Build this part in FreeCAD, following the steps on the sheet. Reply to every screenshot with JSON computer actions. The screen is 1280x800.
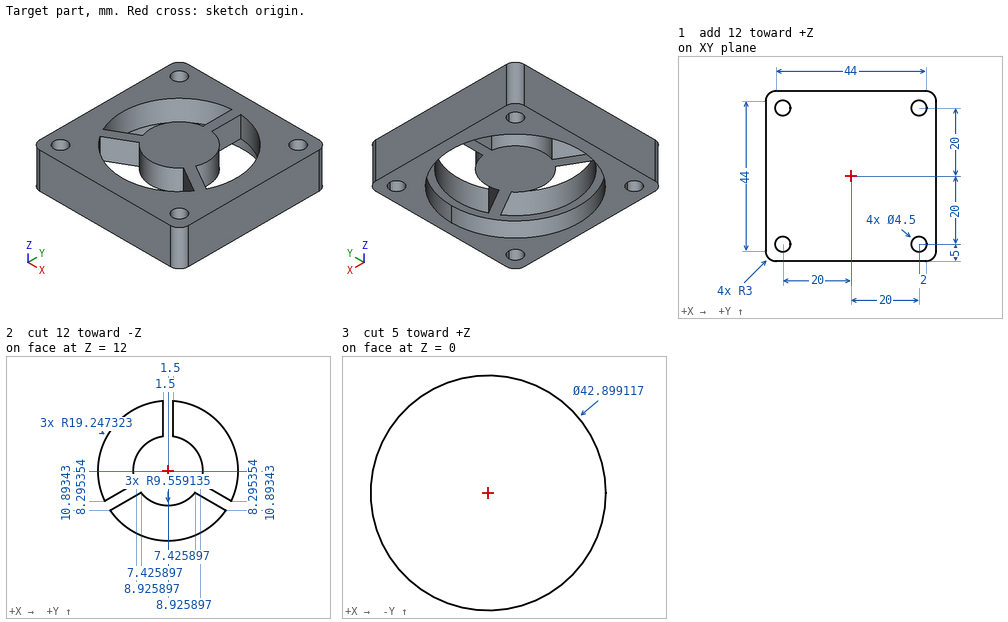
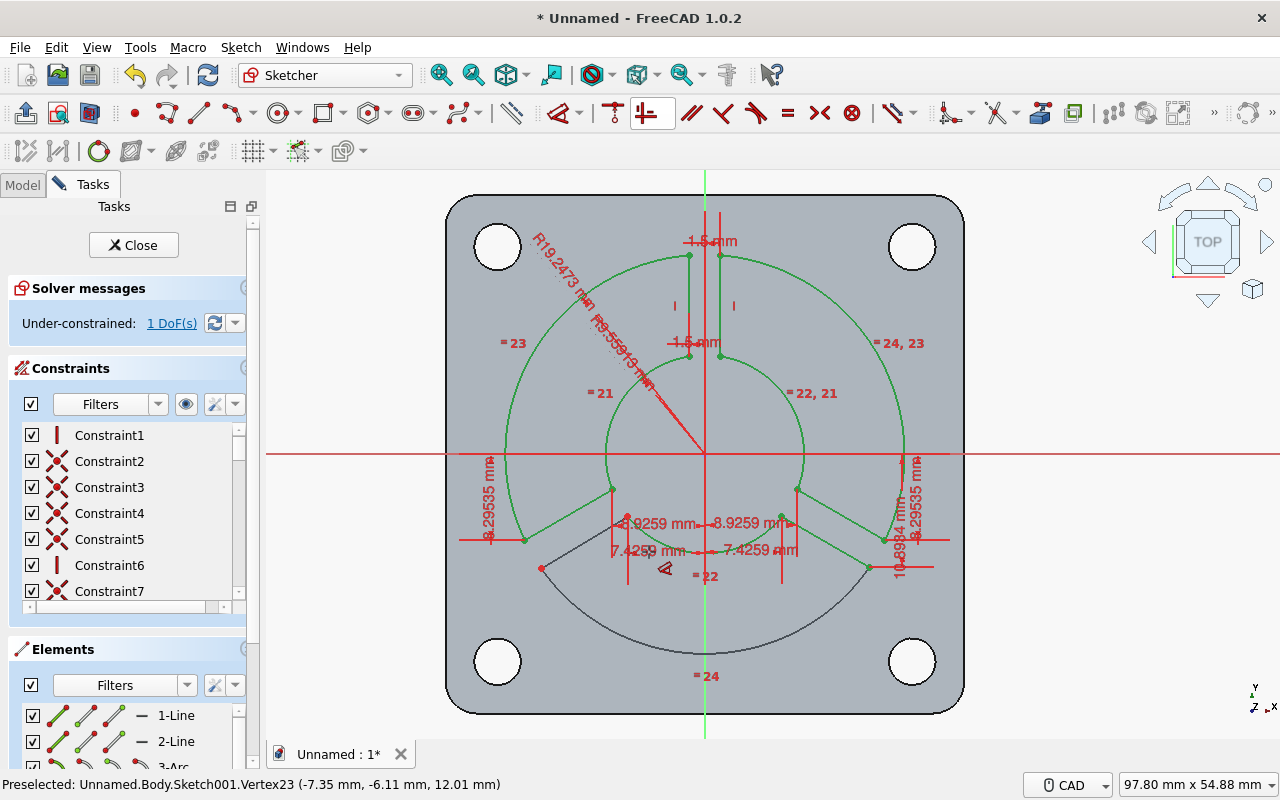
{"action": "left_click", "coordinate": [541, 569]}
{"action": "left_click", "coordinate": [507, 538]}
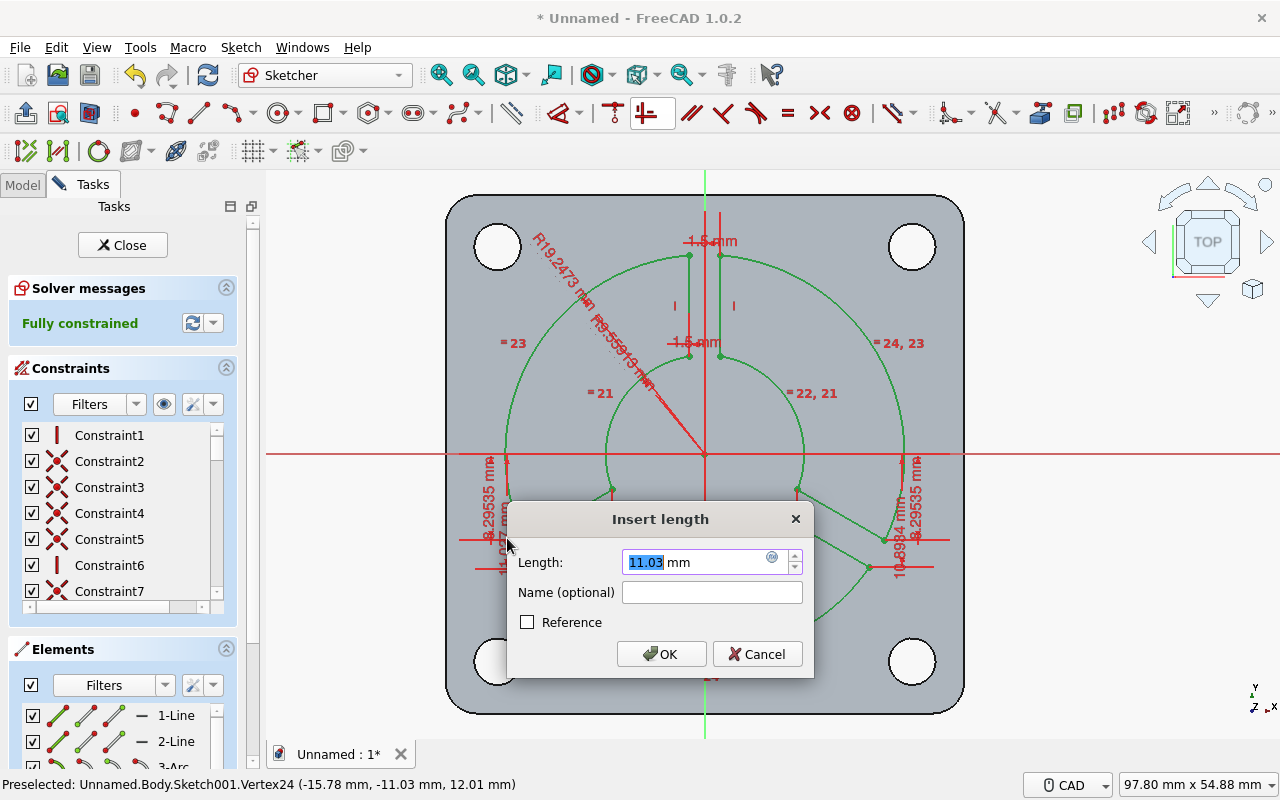
{"action": "type", "text": "10.89343"}
{"action": "key", "text": "Return"}
{"action": "key", "text": "Escape"}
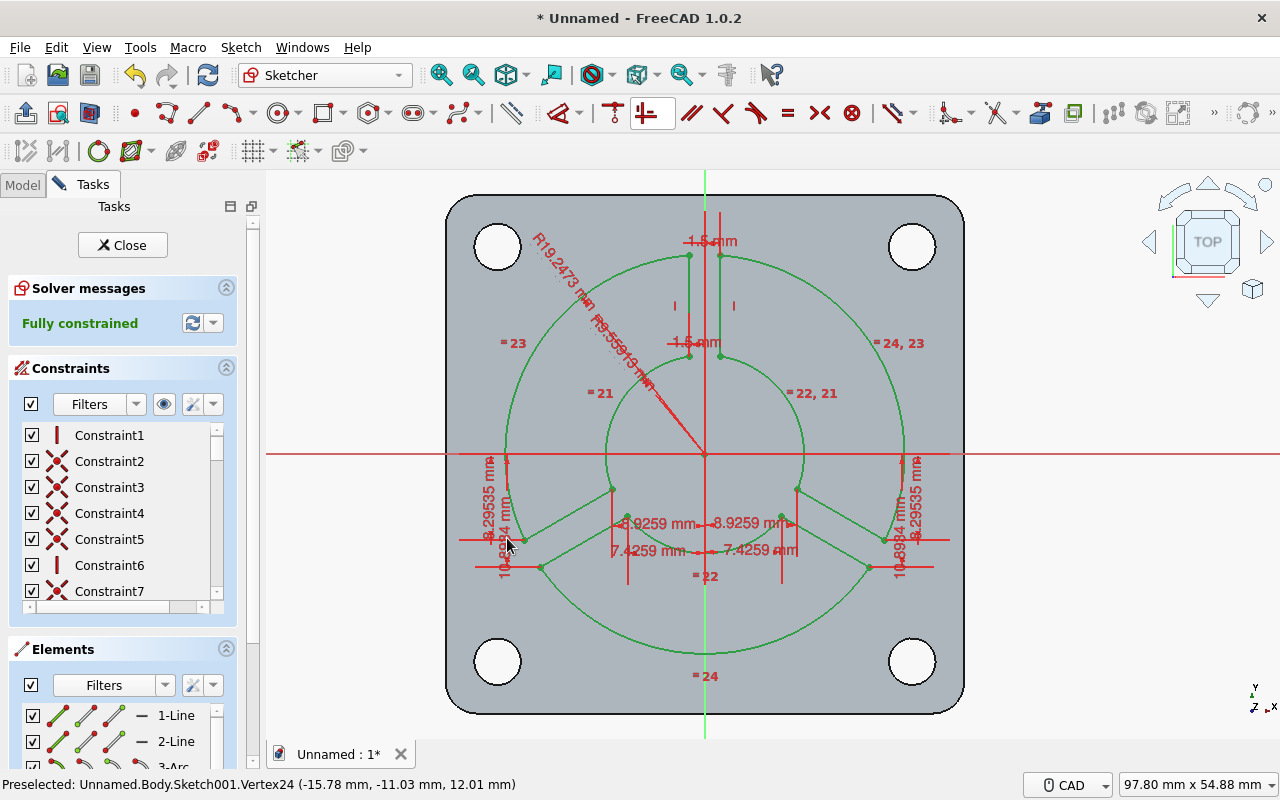
{"action": "left_click", "coordinate": [123, 245]}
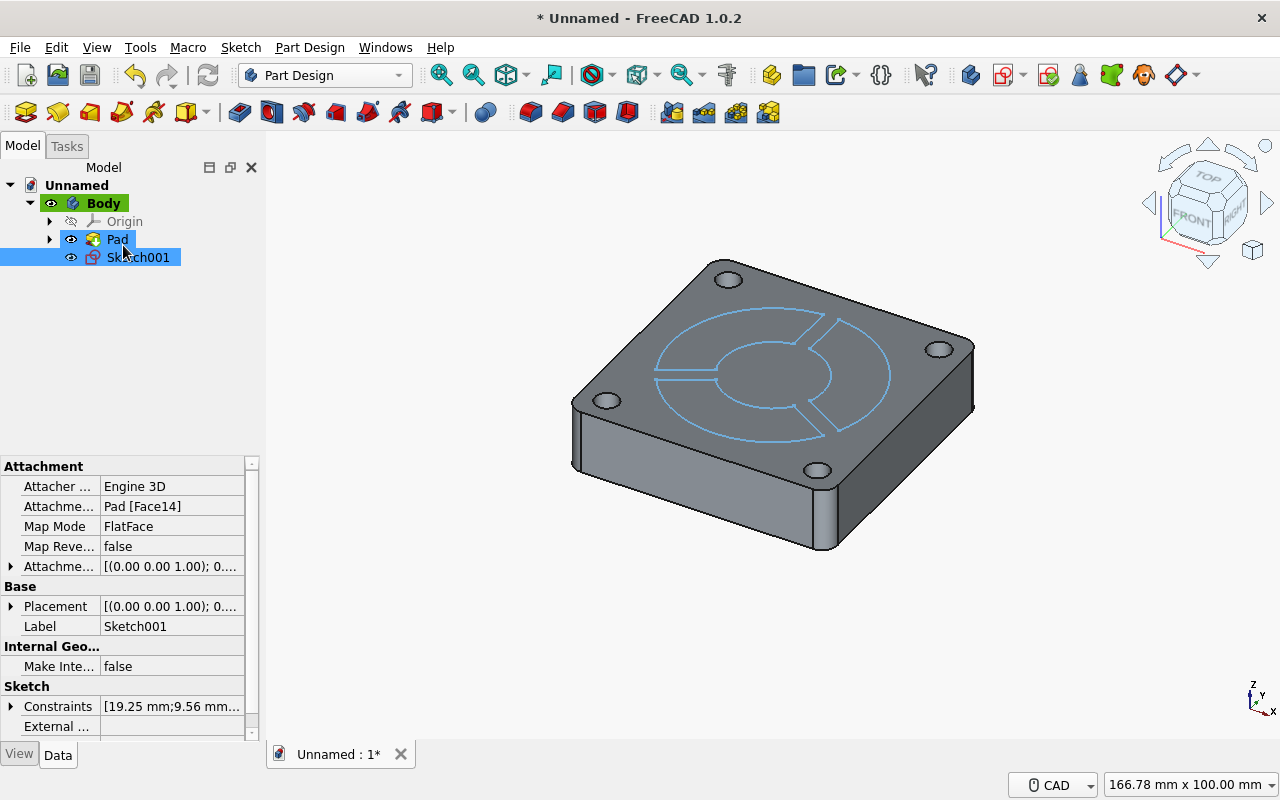
{"action": "left_click", "coordinate": [240, 112]}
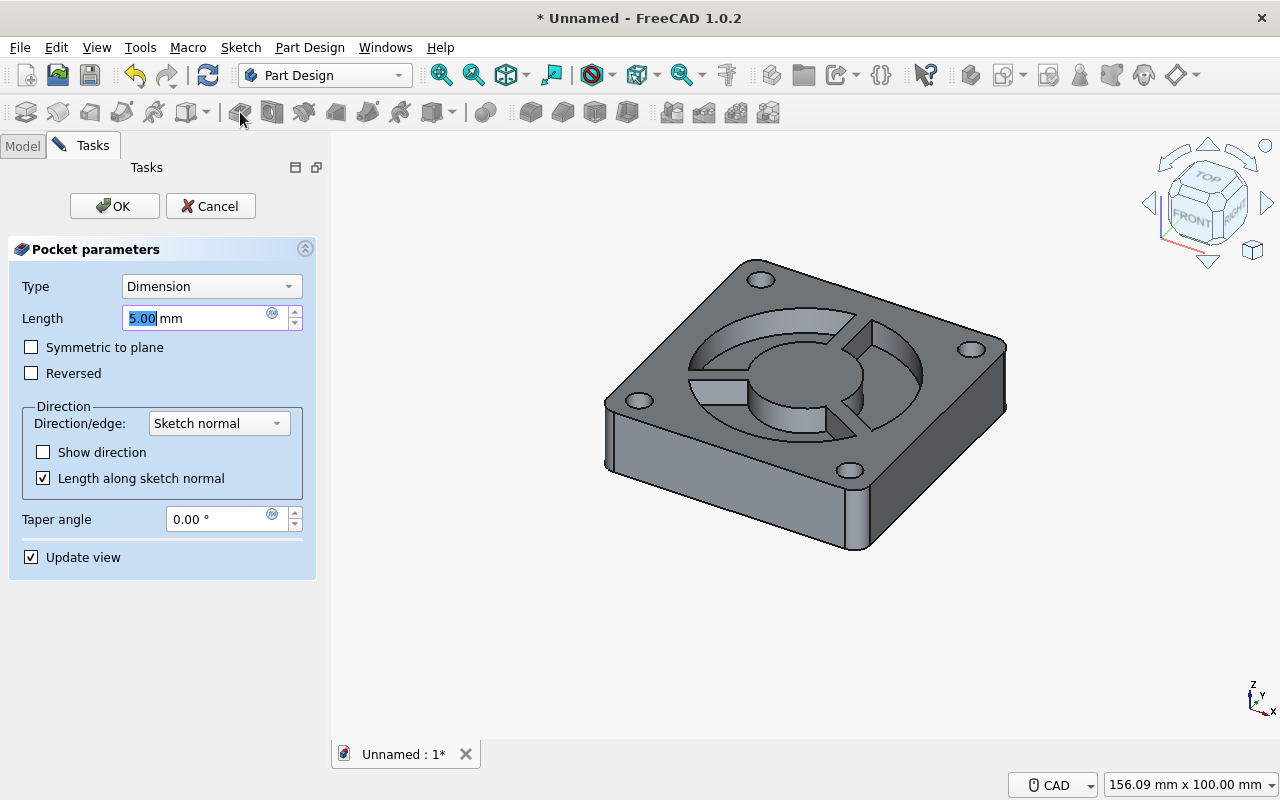
{"action": "type", "text": "12"}
{"action": "key", "text": "Tab"}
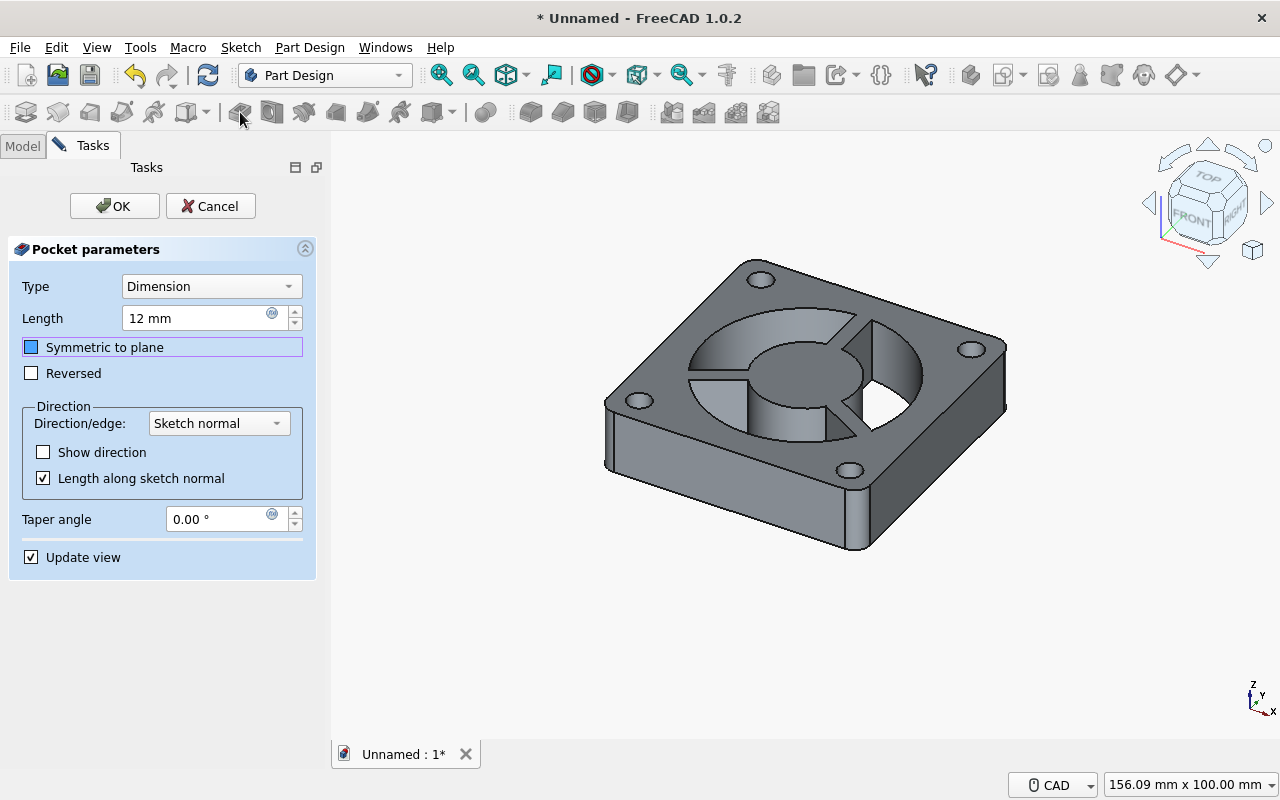
{"action": "left_click", "coordinate": [115, 206]}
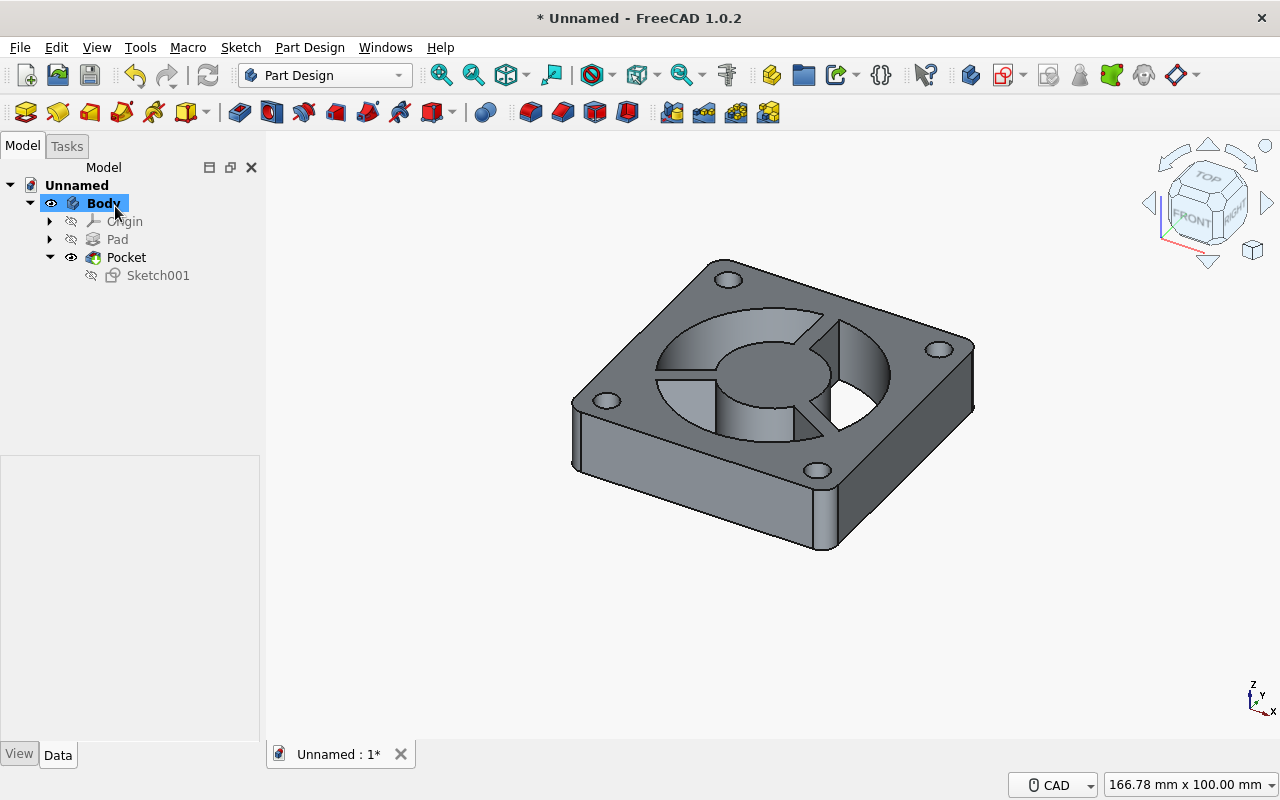
{"action": "key", "text": "5"}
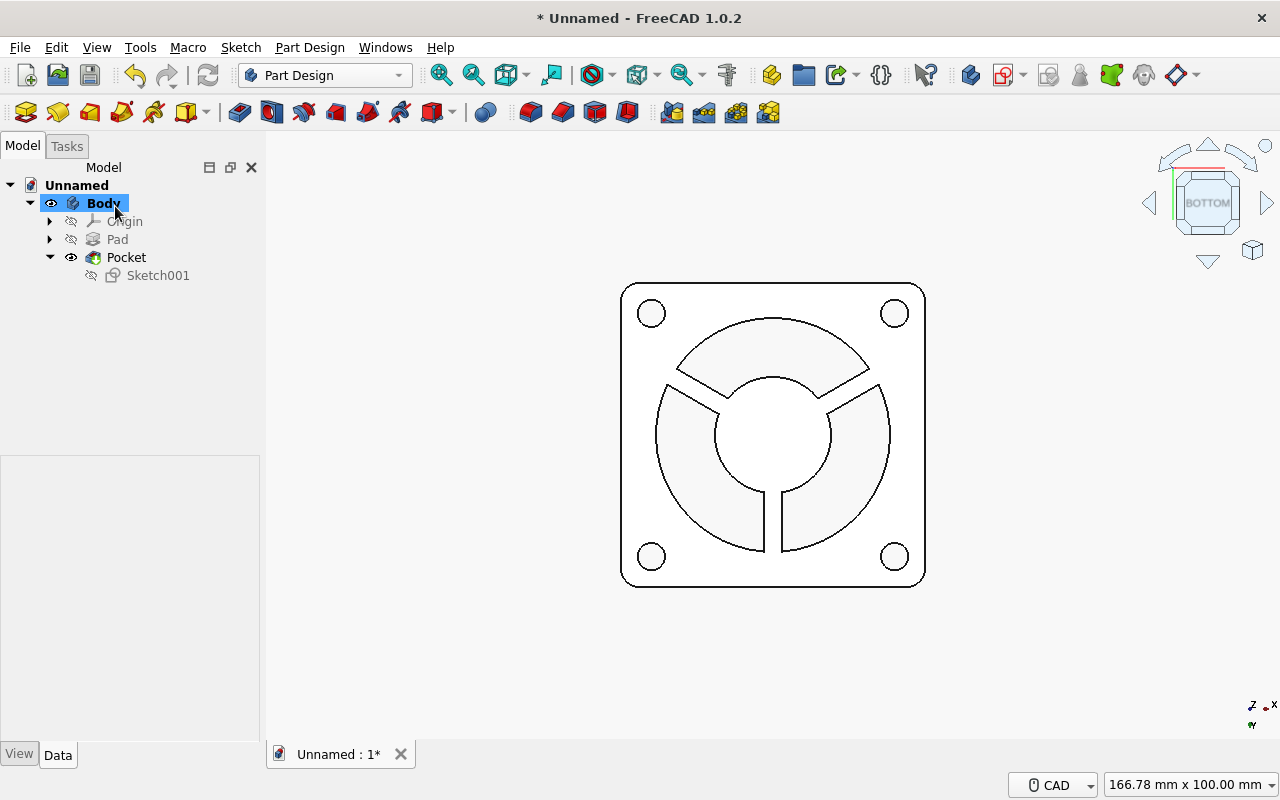
{"action": "left_click", "coordinate": [773, 434]}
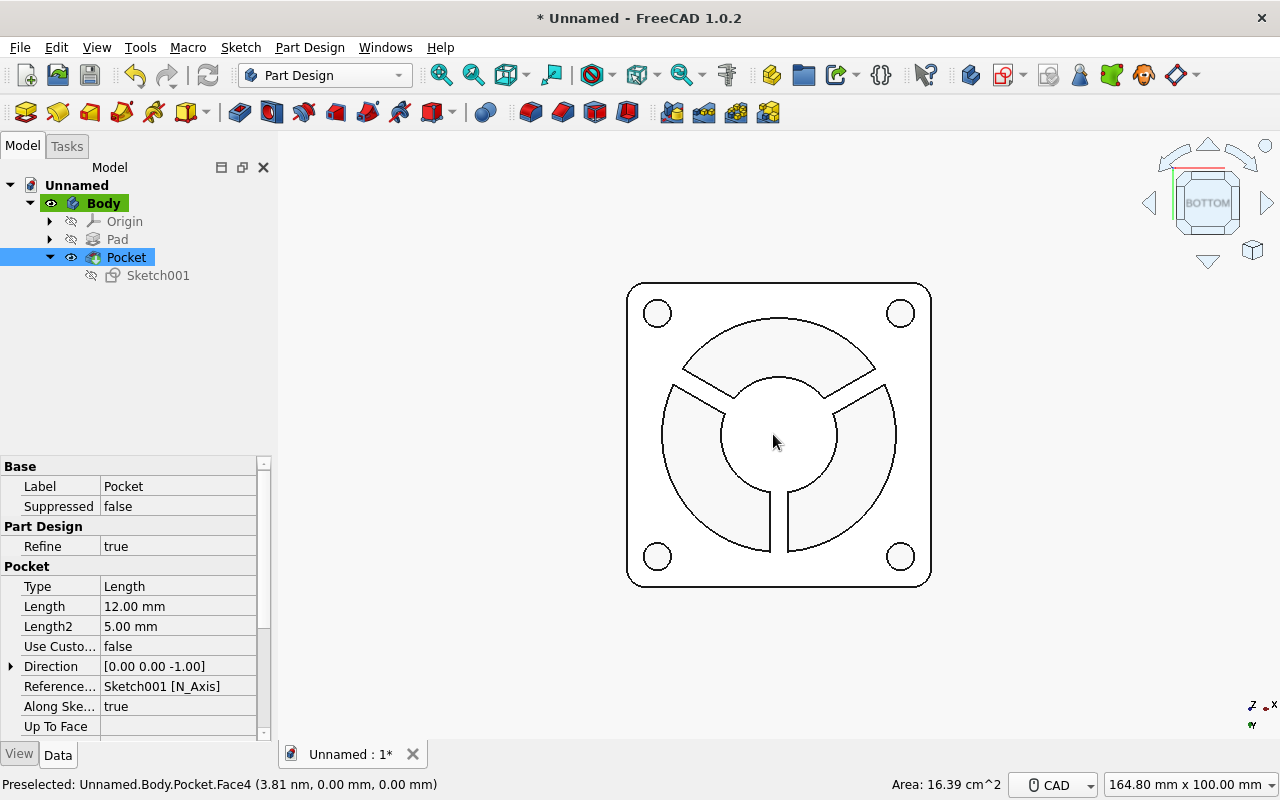
{"action": "left_click", "coordinate": [1004, 76]}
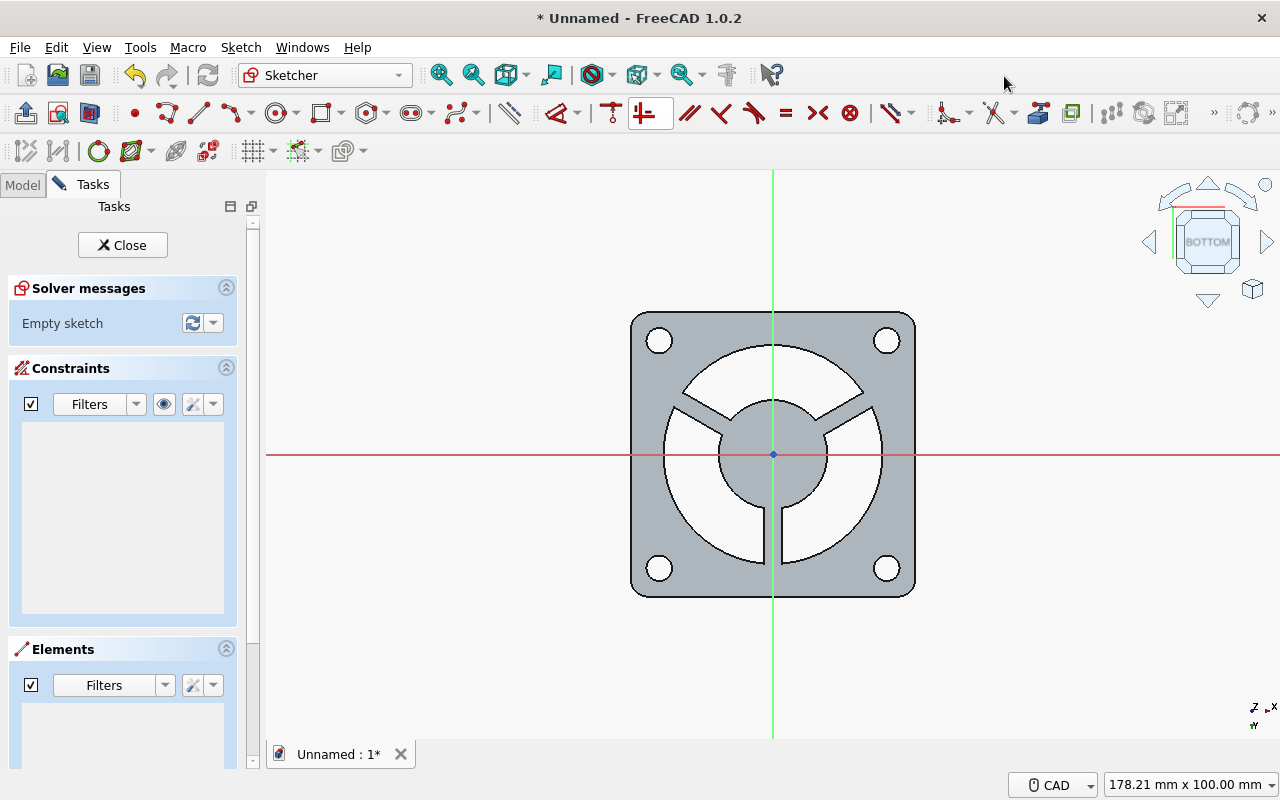
{"action": "scroll", "coordinate": [912, 455], "scroll_direction": "up", "scroll_amount": 2}